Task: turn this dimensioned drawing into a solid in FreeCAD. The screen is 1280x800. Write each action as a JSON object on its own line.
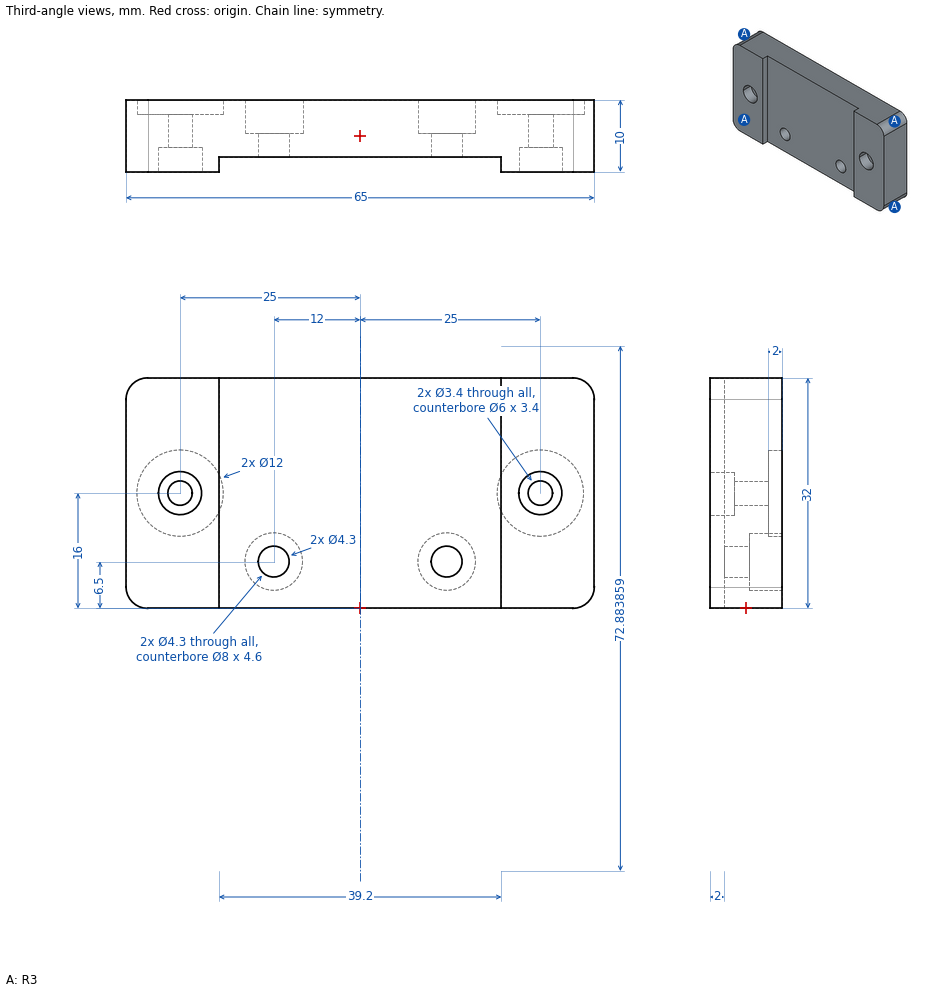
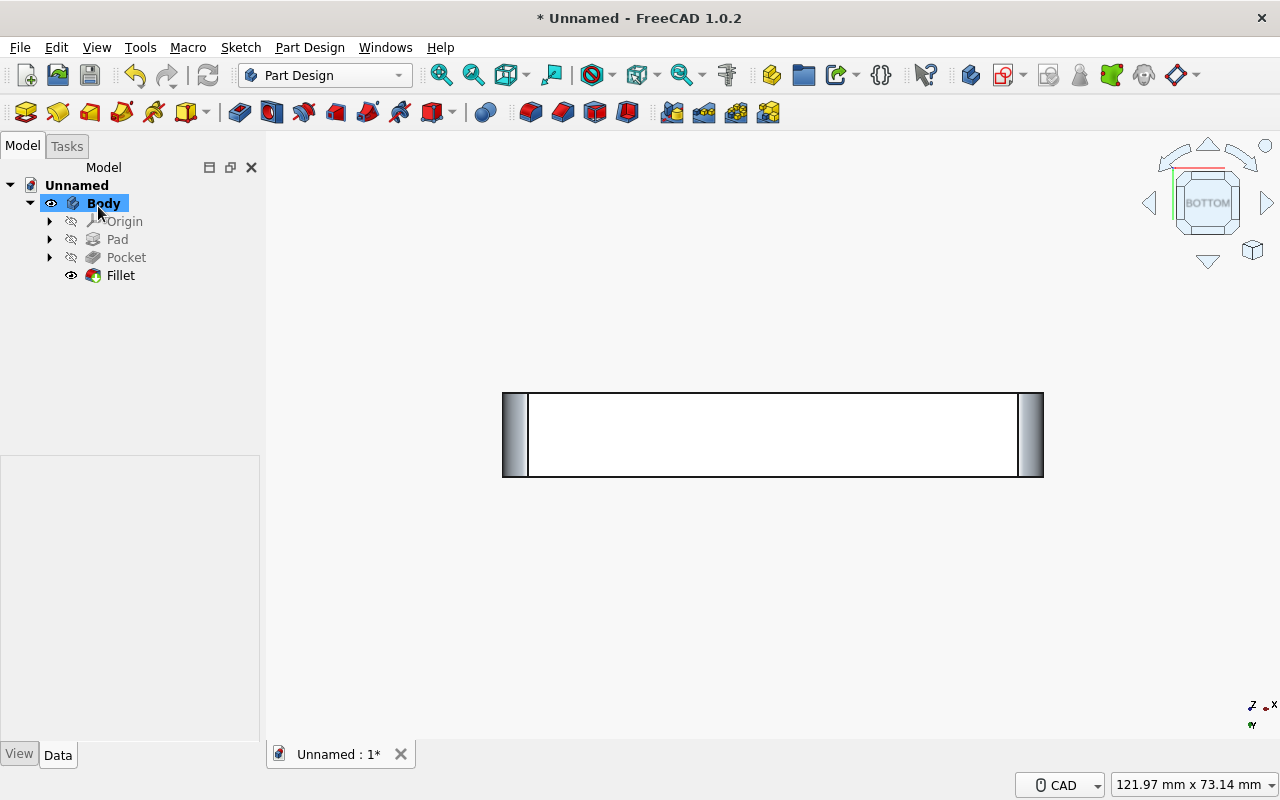
{"action": "key", "text": "4"}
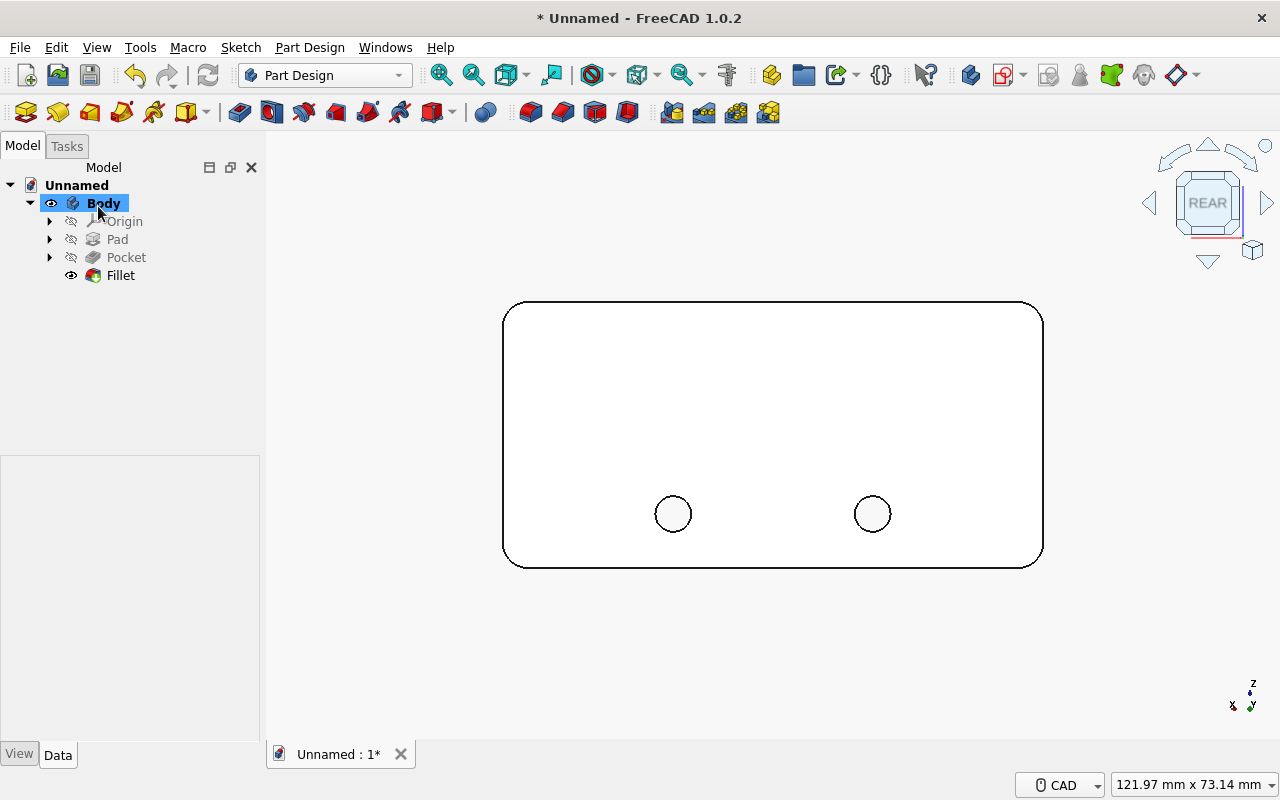
{"action": "left_click", "coordinate": [773, 434]}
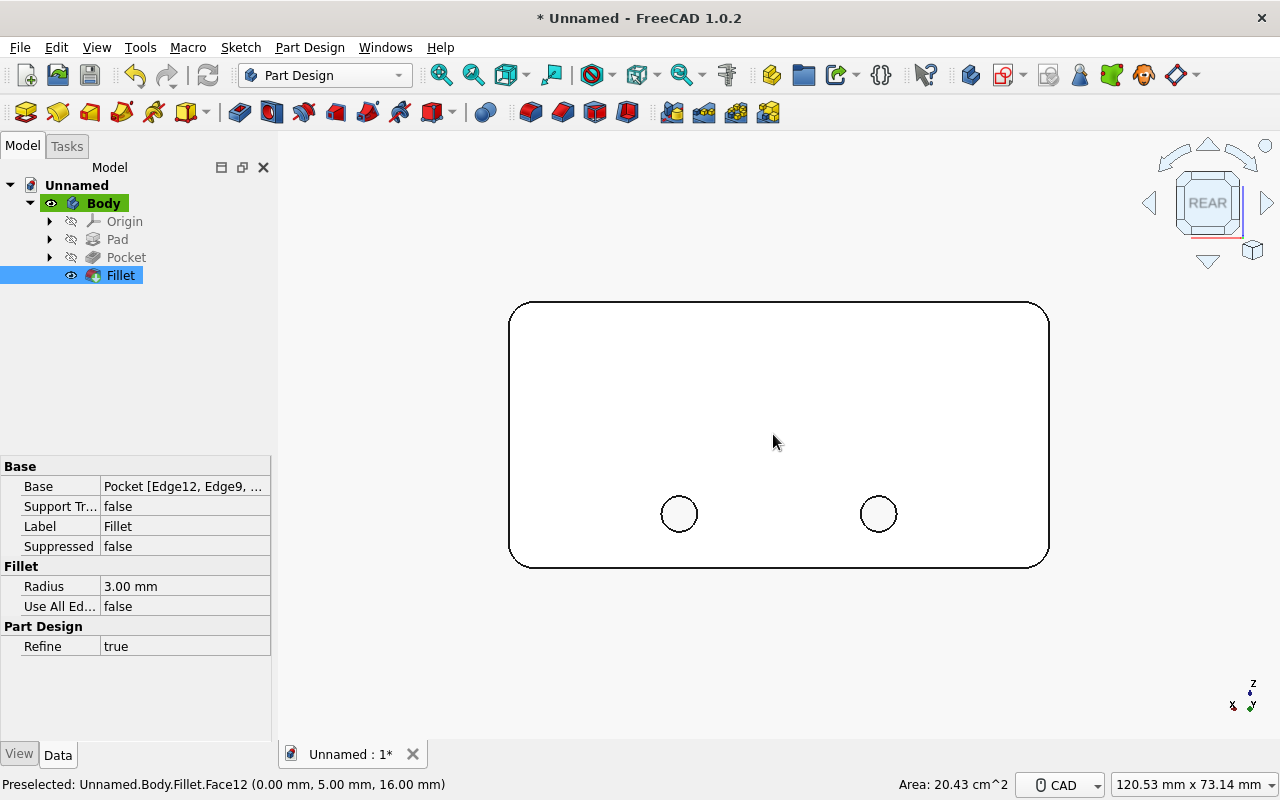
{"action": "left_click", "coordinate": [1004, 76]}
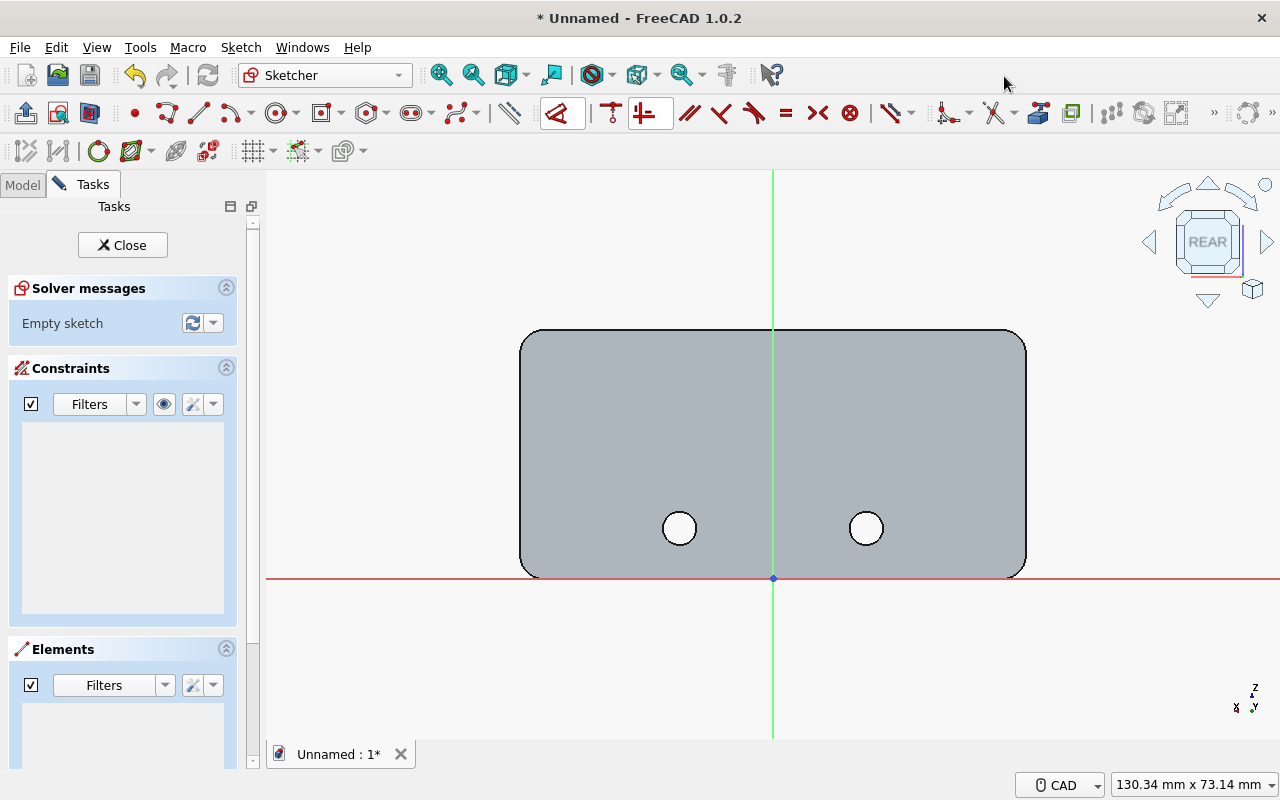
{"action": "left_click", "coordinate": [276, 114]}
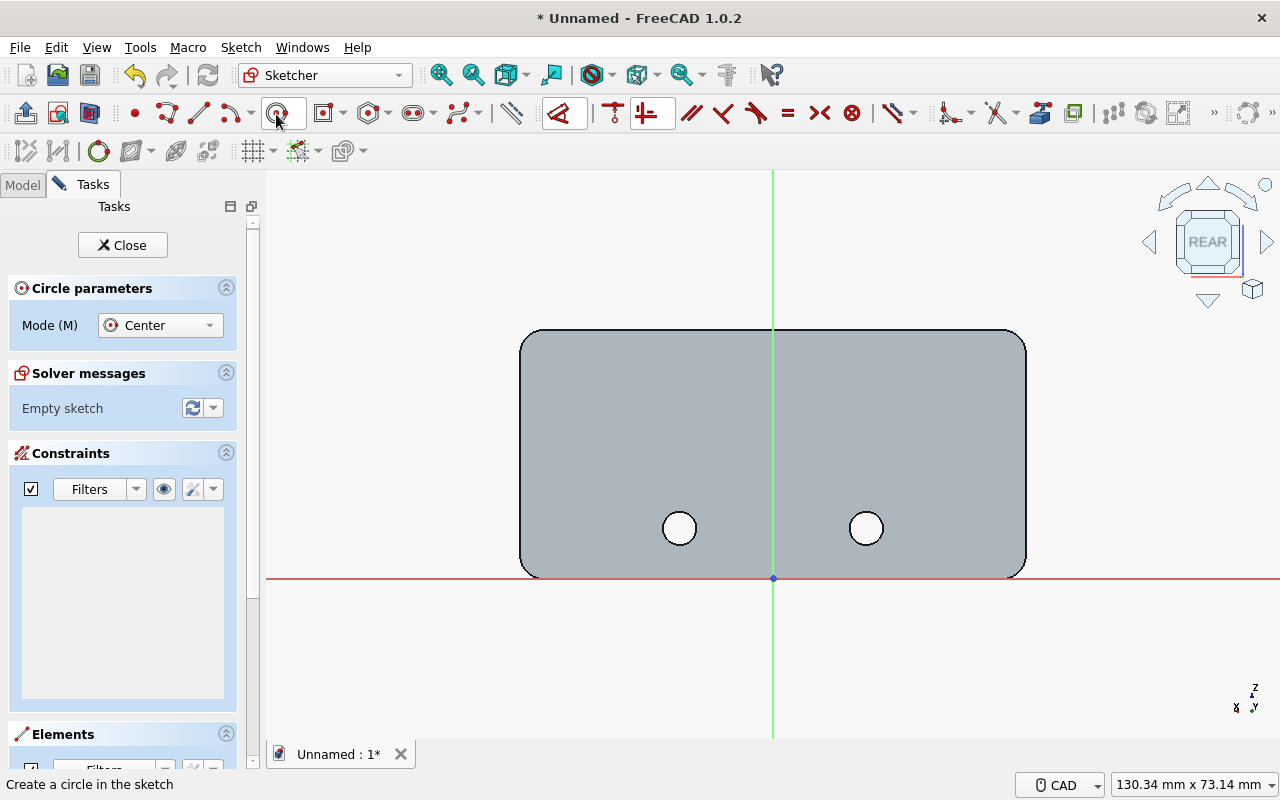
{"action": "left_click", "coordinate": [967, 455]}
{"action": "left_click", "coordinate": [1001, 421]}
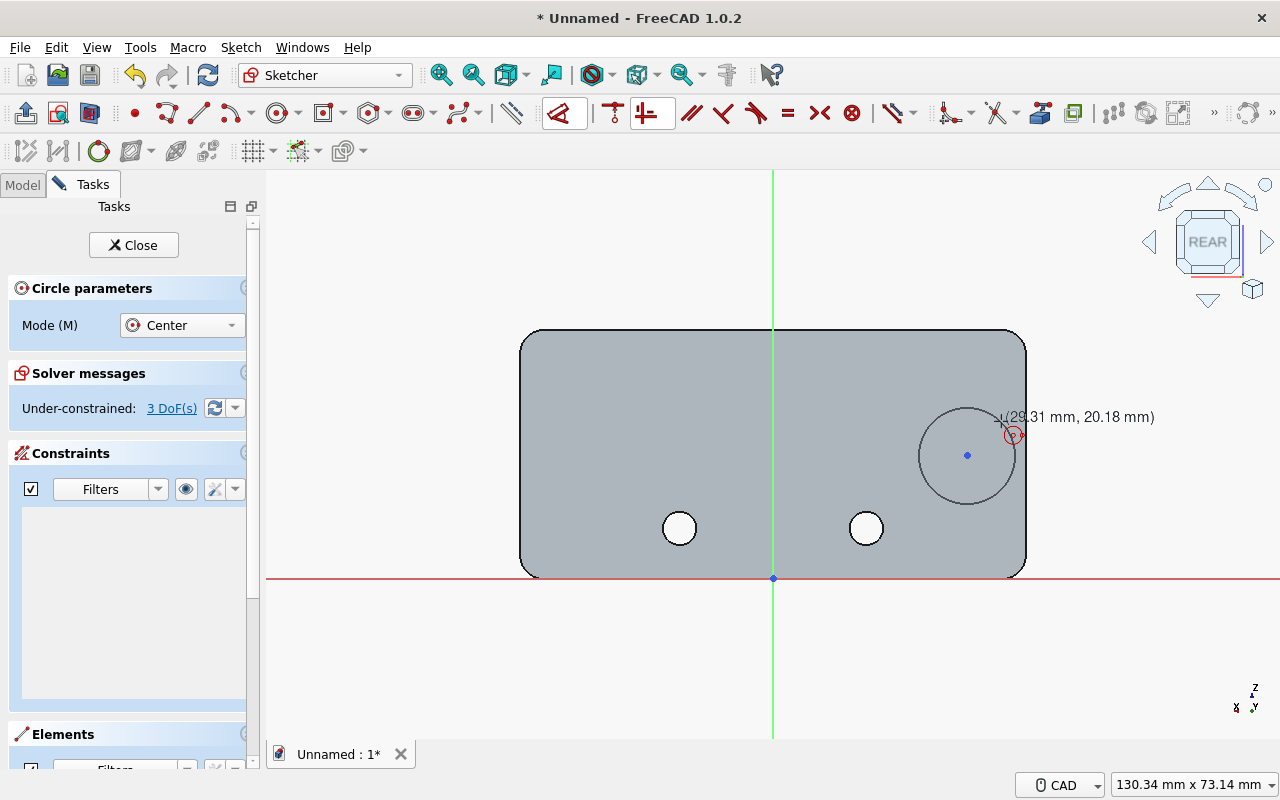
{"action": "left_click", "coordinate": [579, 455]}
{"action": "left_click", "coordinate": [612, 421]}
{"action": "key", "text": "Escape"}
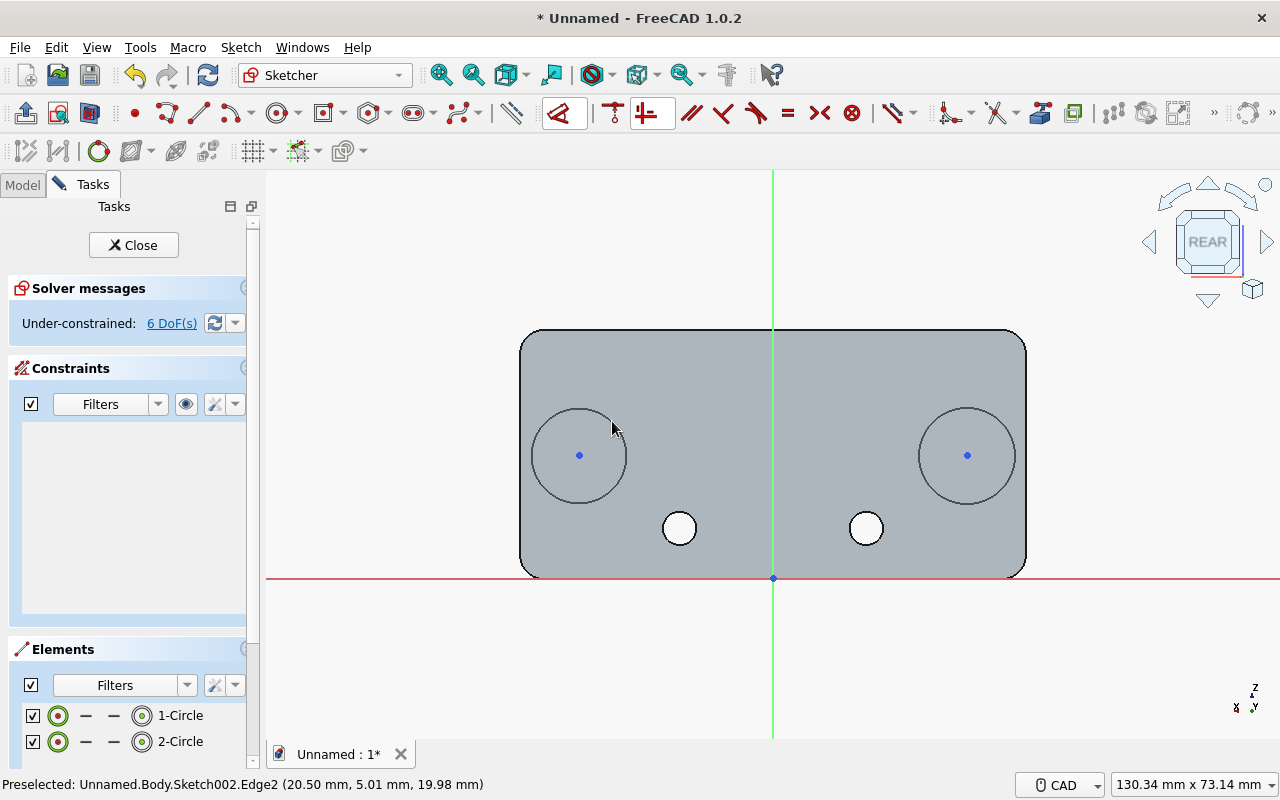
{"action": "left_click", "coordinate": [1001, 422]}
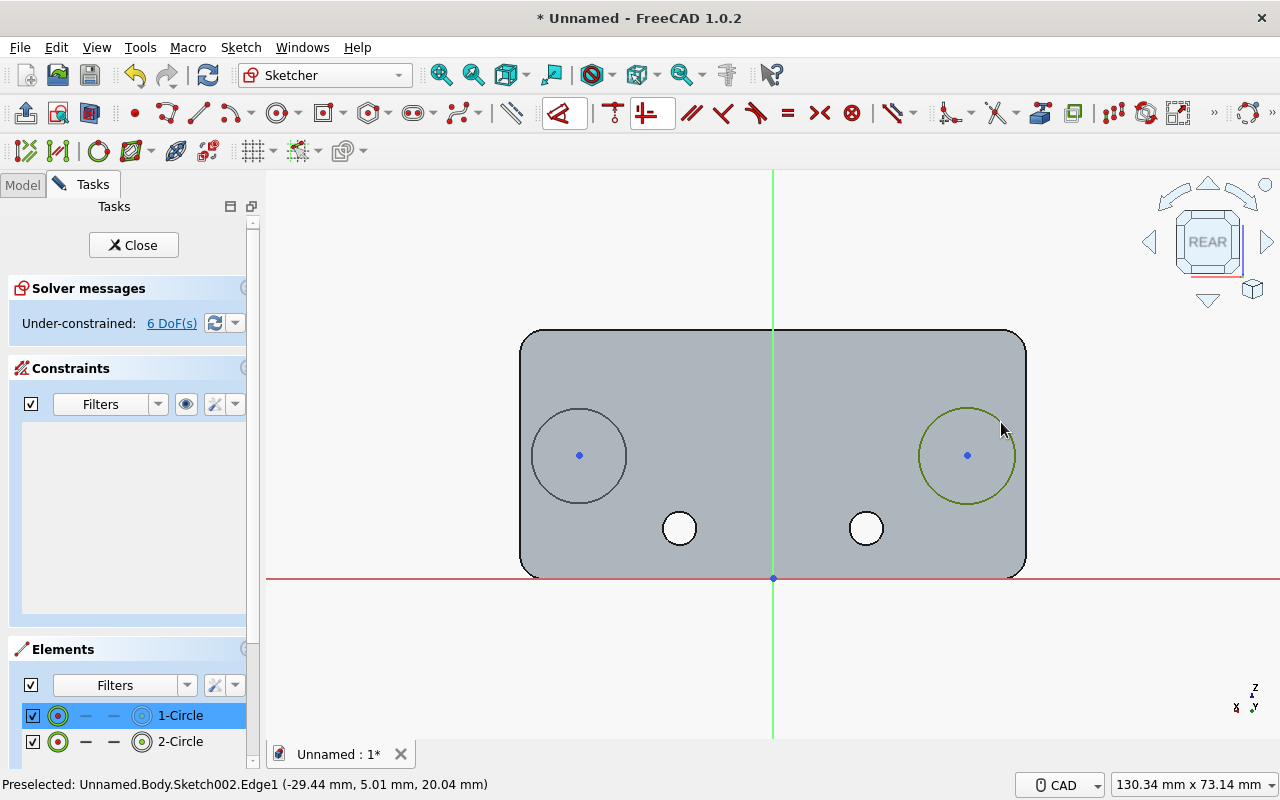
{"action": "left_click", "coordinate": [612, 422]}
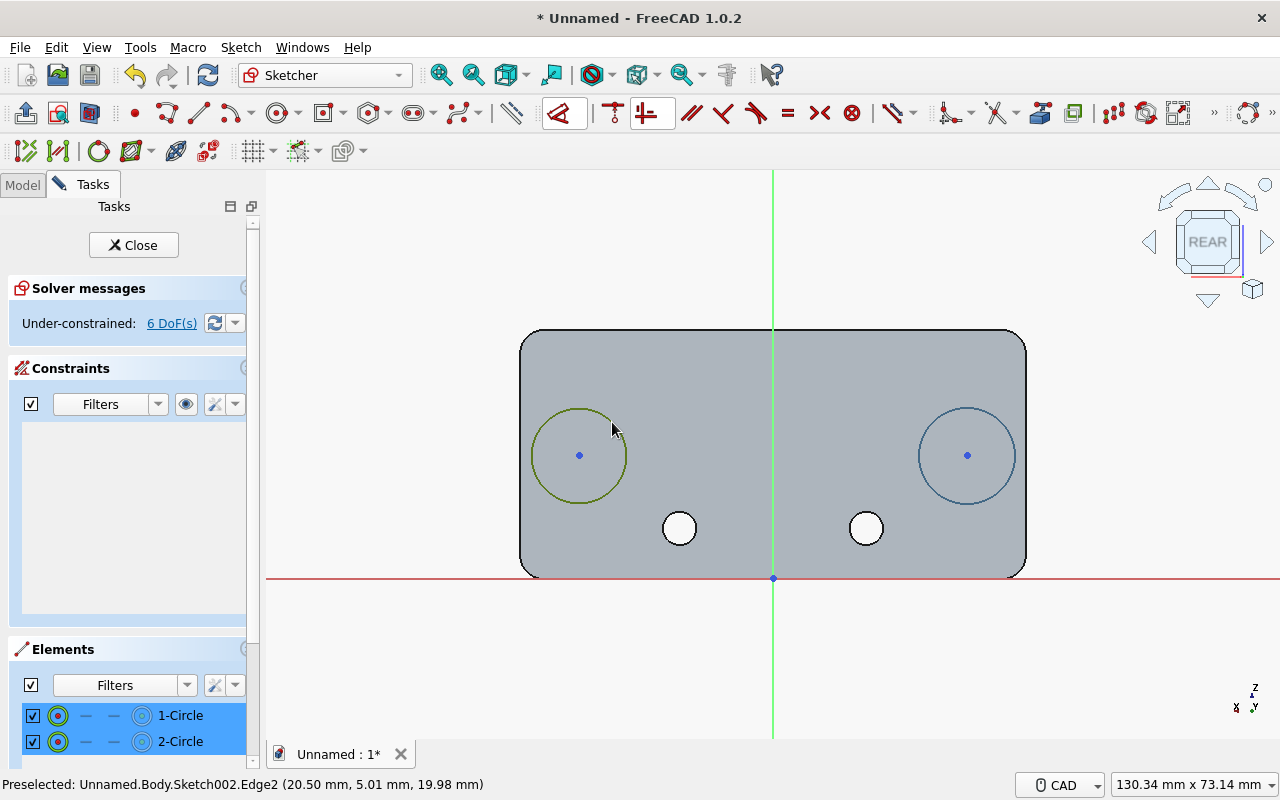
{"action": "left_click", "coordinate": [788, 114]}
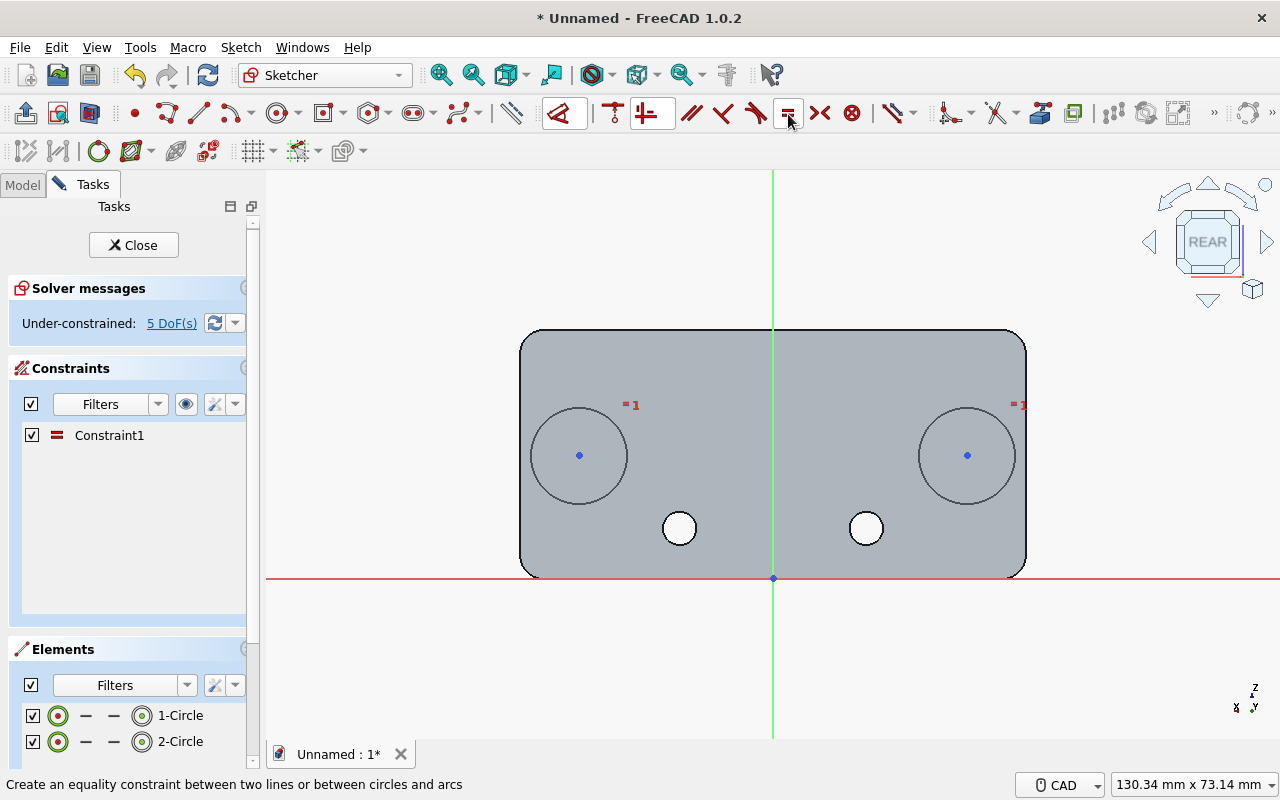
{"action": "left_click", "coordinate": [967, 456]}